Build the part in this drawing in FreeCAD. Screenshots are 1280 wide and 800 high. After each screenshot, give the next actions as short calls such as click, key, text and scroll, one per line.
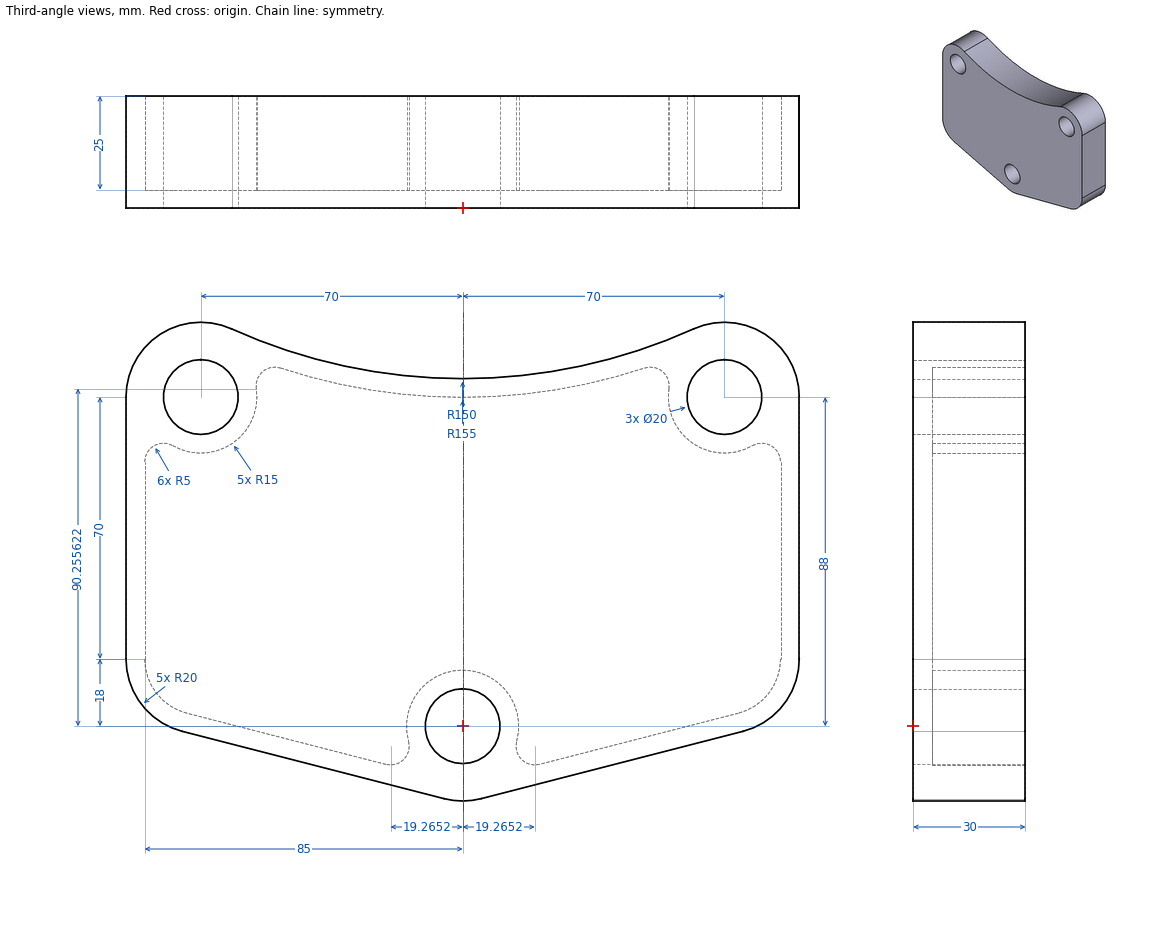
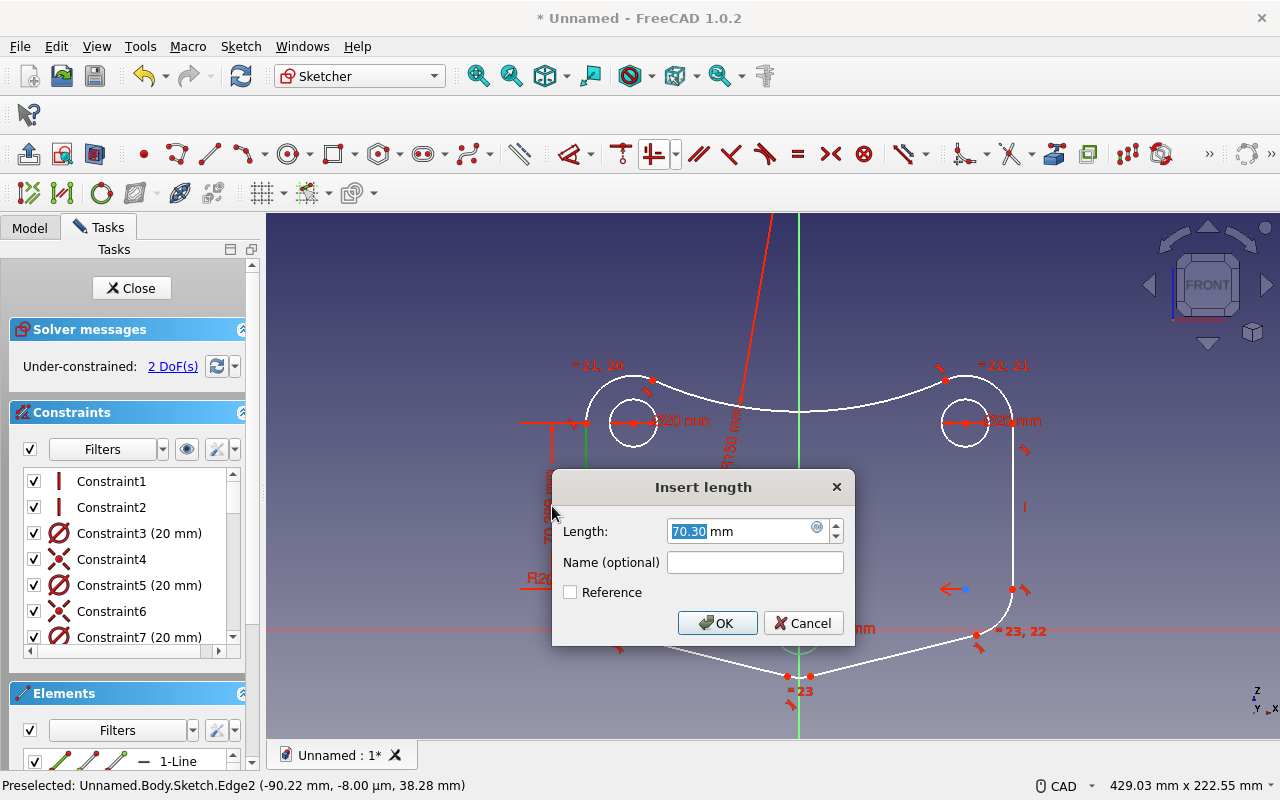
text(70)
key(Return)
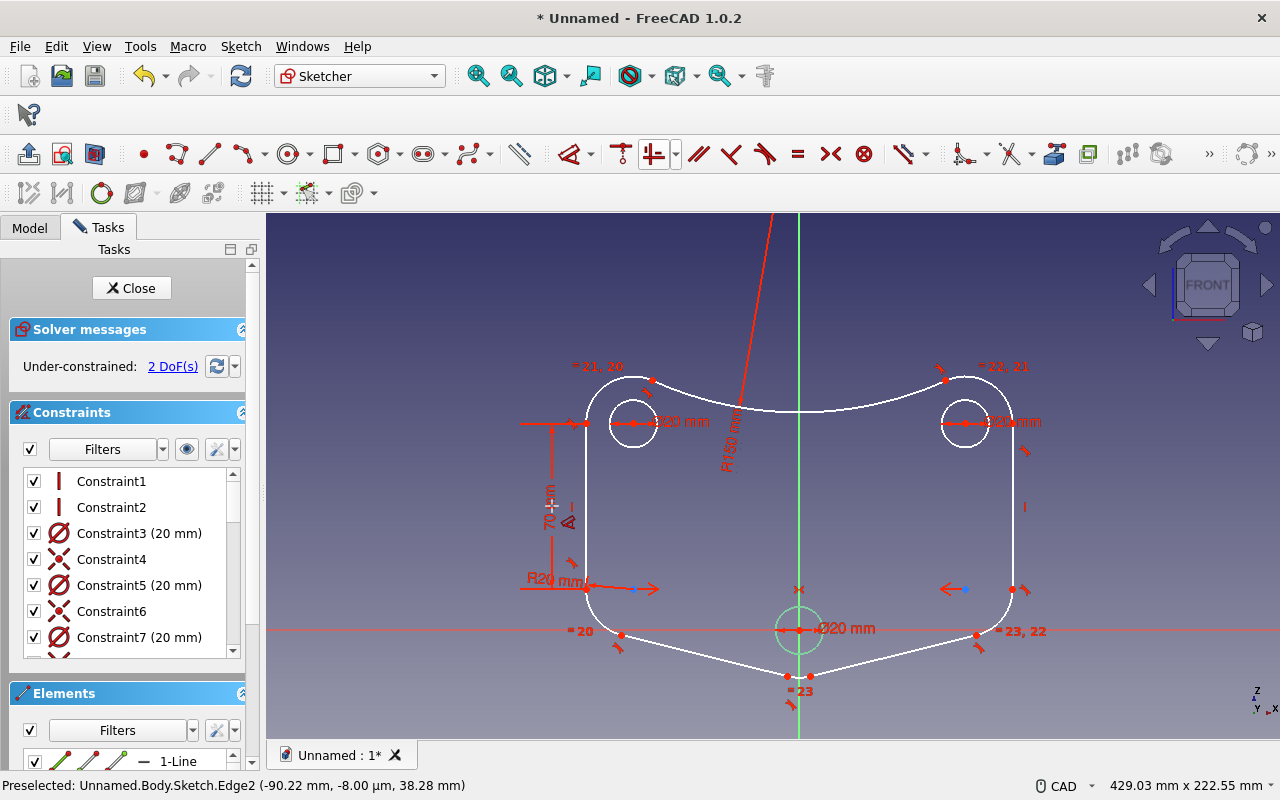
click(965, 424)
click(844, 390)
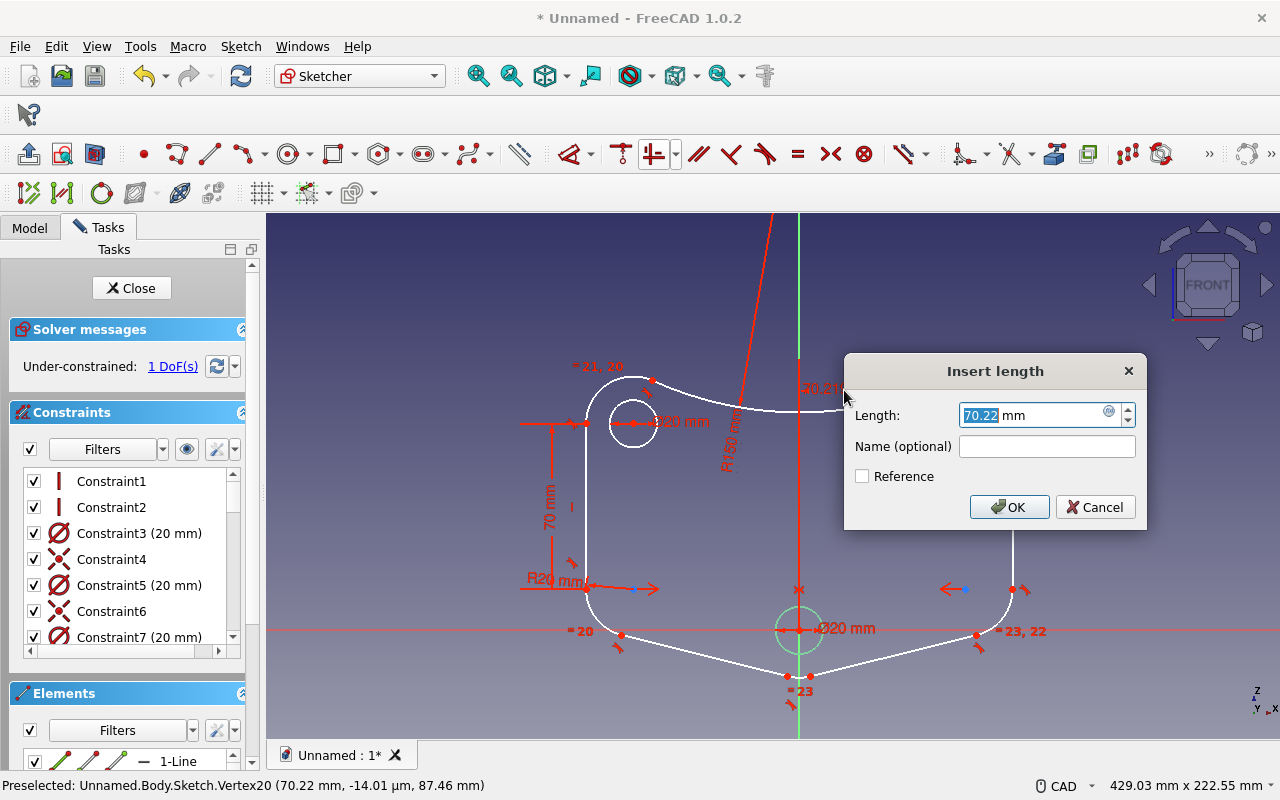
text(70)
key(Return)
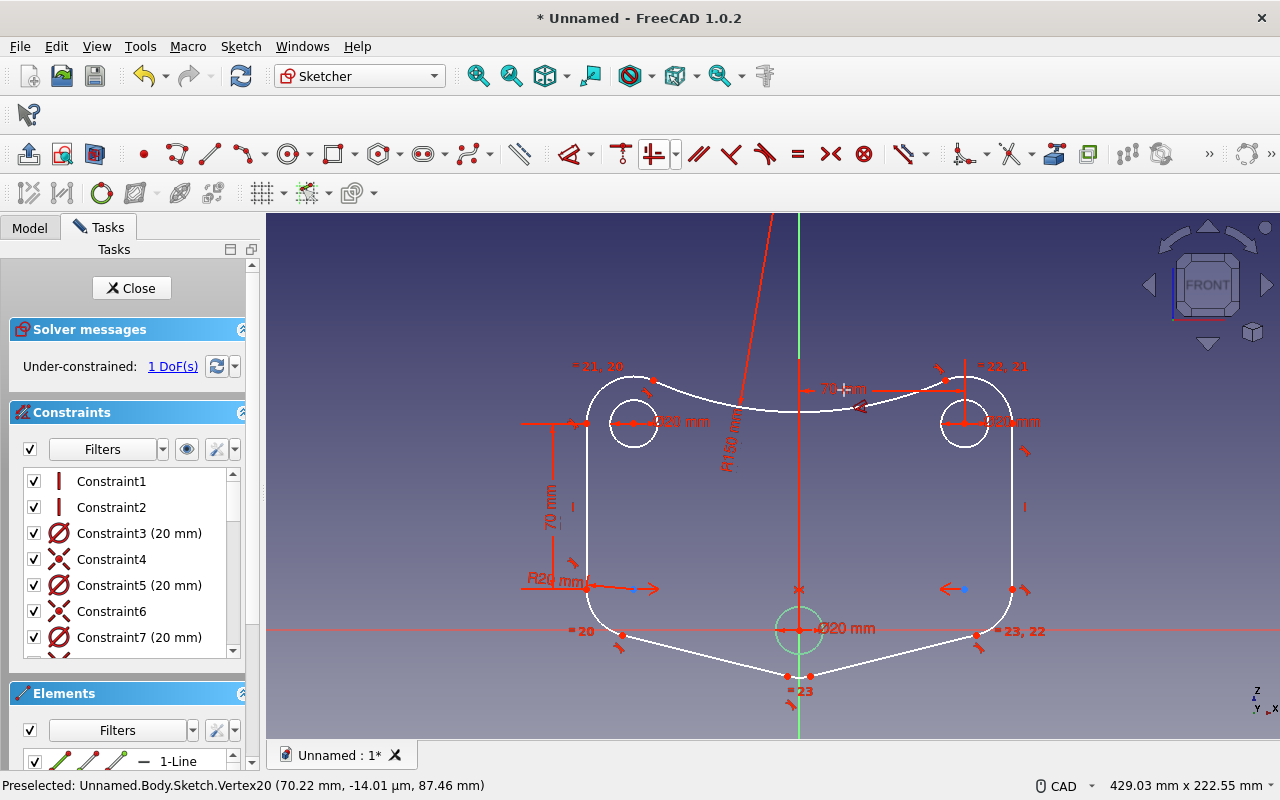
click(965, 424)
click(999, 527)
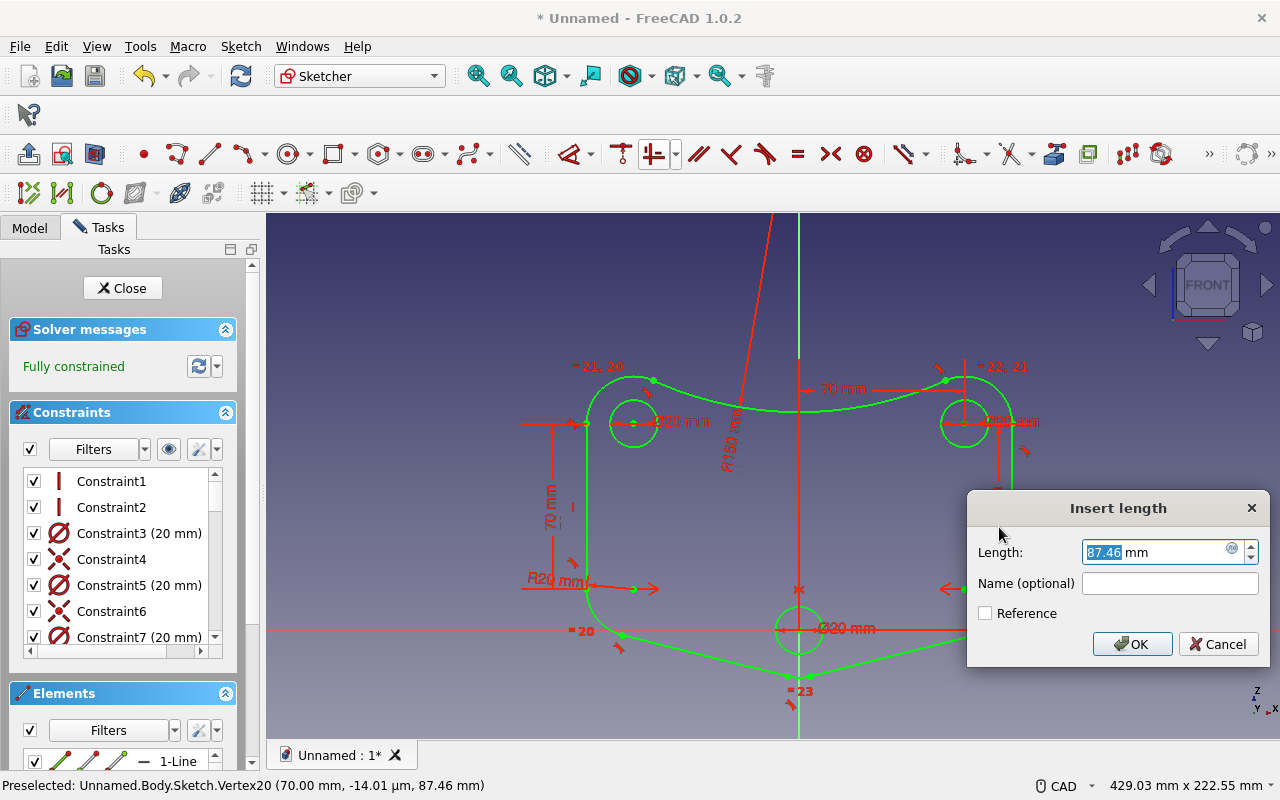
text(88)
key(Return)
key(Escape)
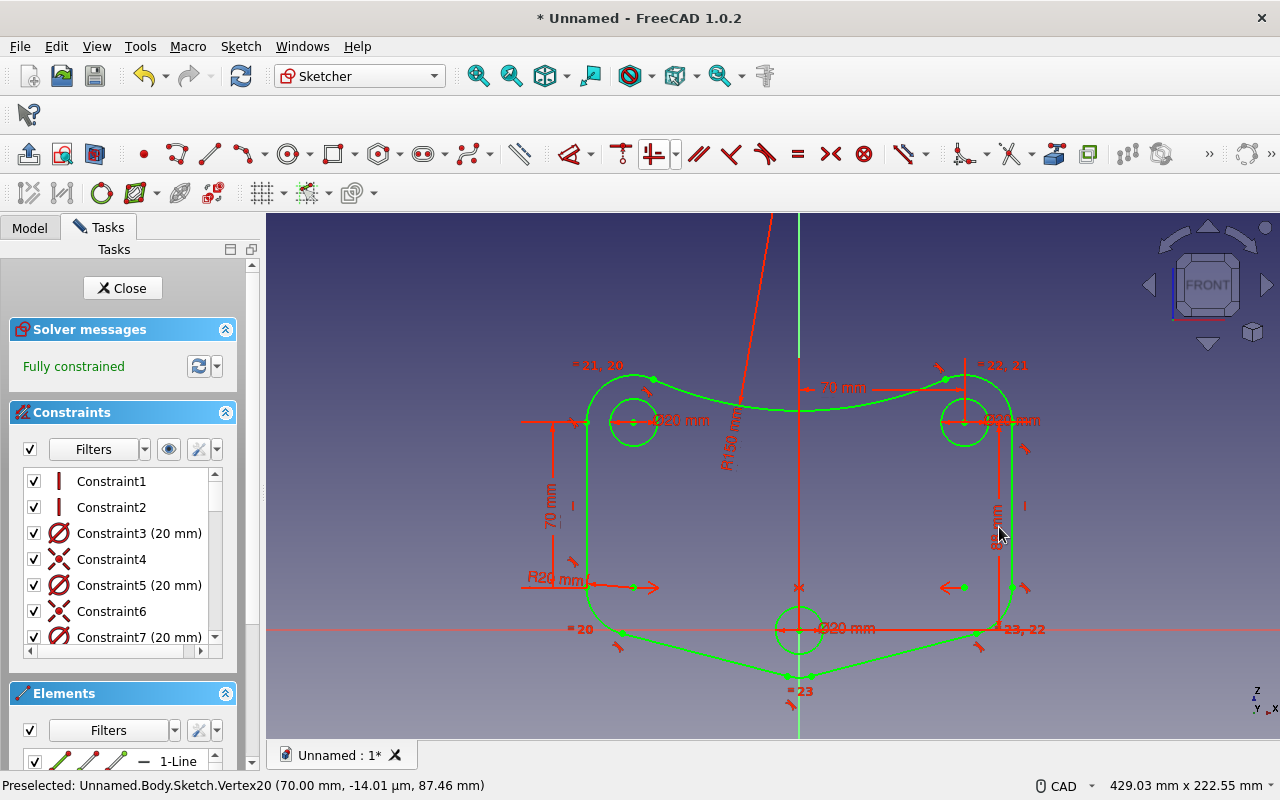
click(123, 288)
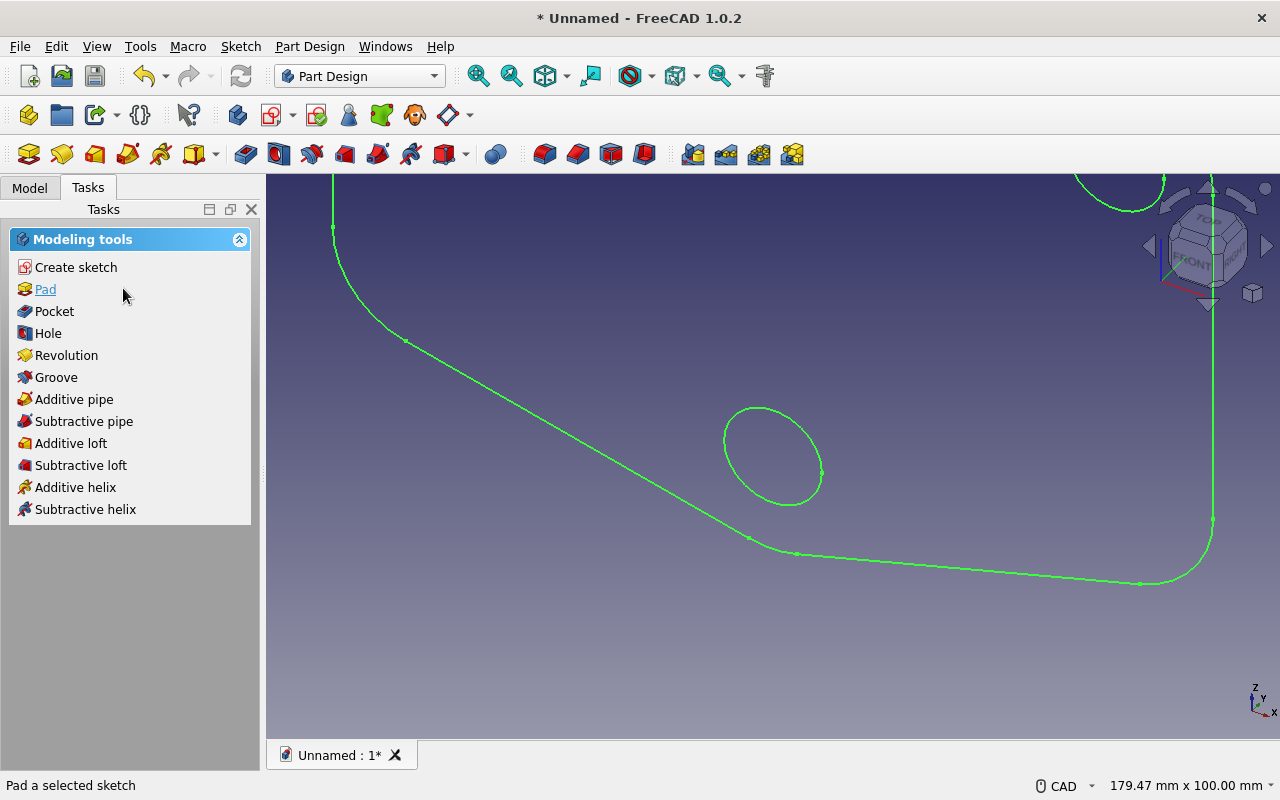
click(29, 154)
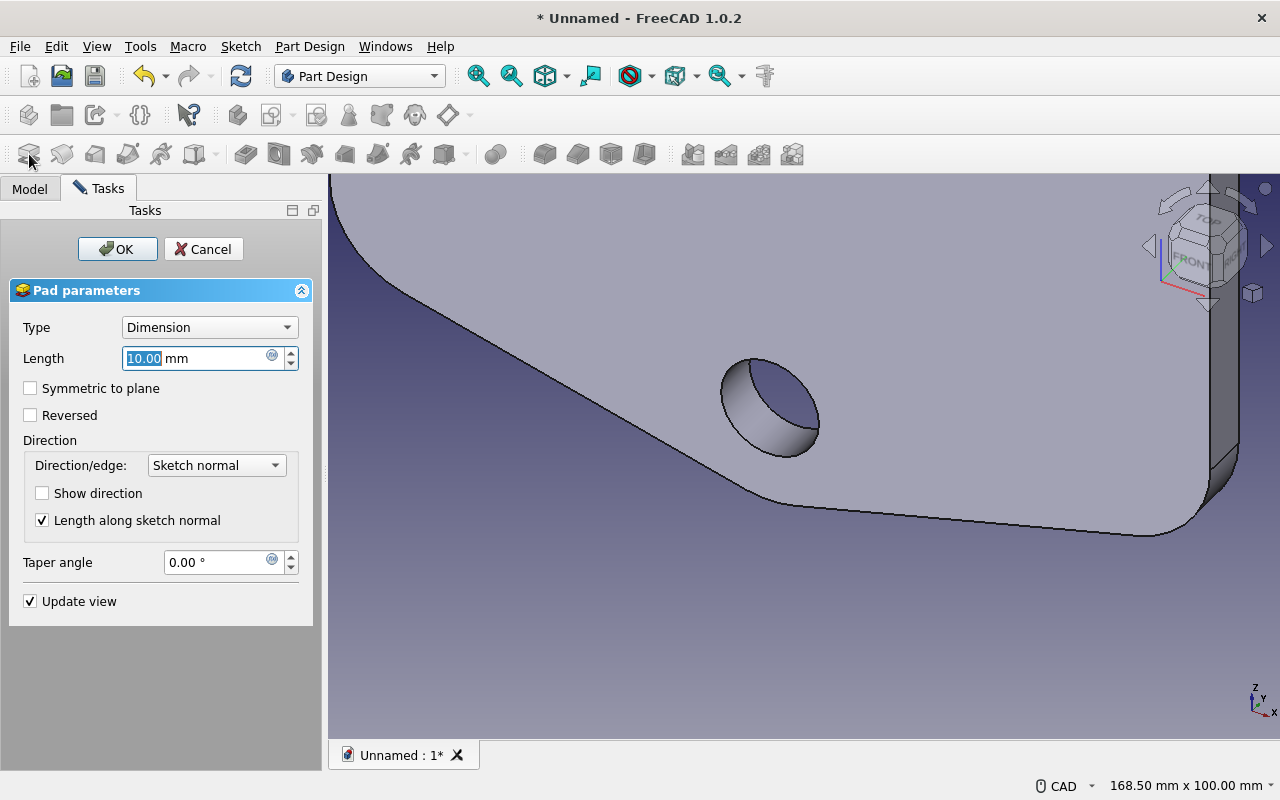
text(30)
key(Tab)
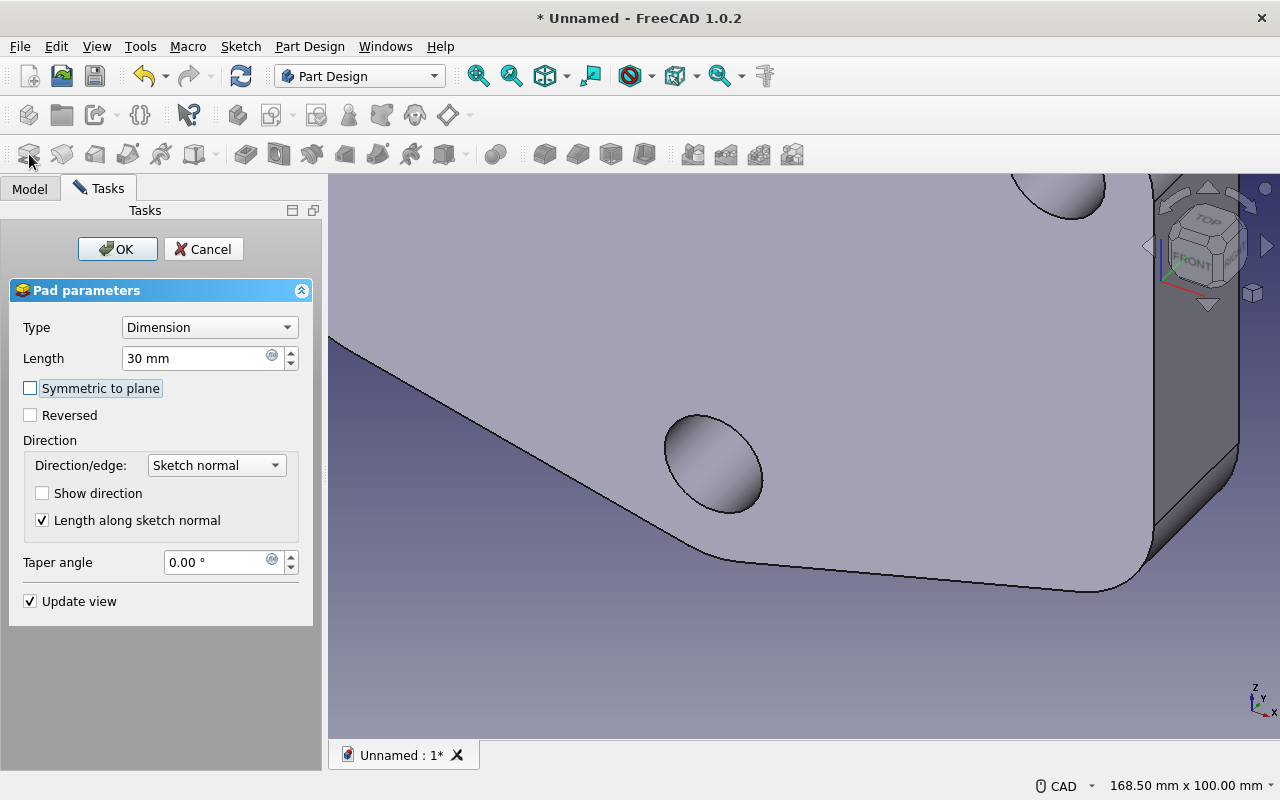
click(31, 415)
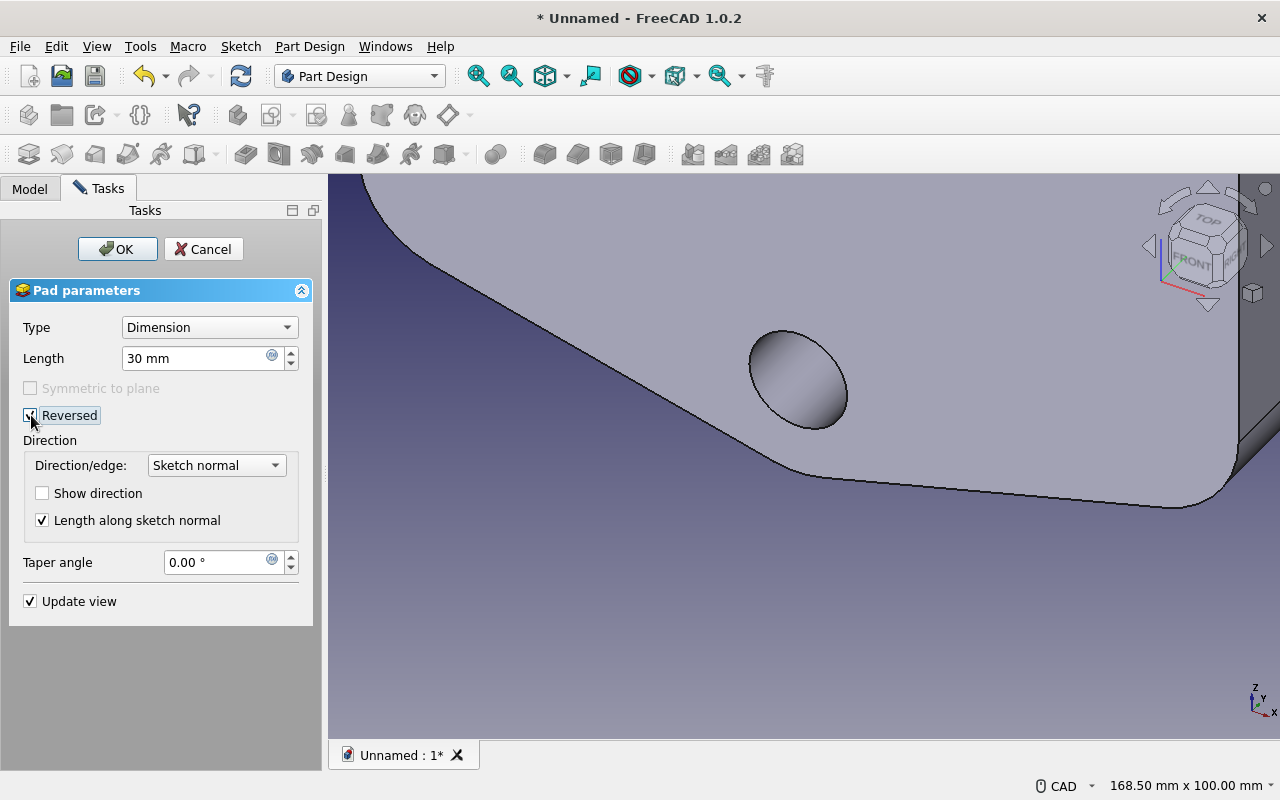
click(118, 249)